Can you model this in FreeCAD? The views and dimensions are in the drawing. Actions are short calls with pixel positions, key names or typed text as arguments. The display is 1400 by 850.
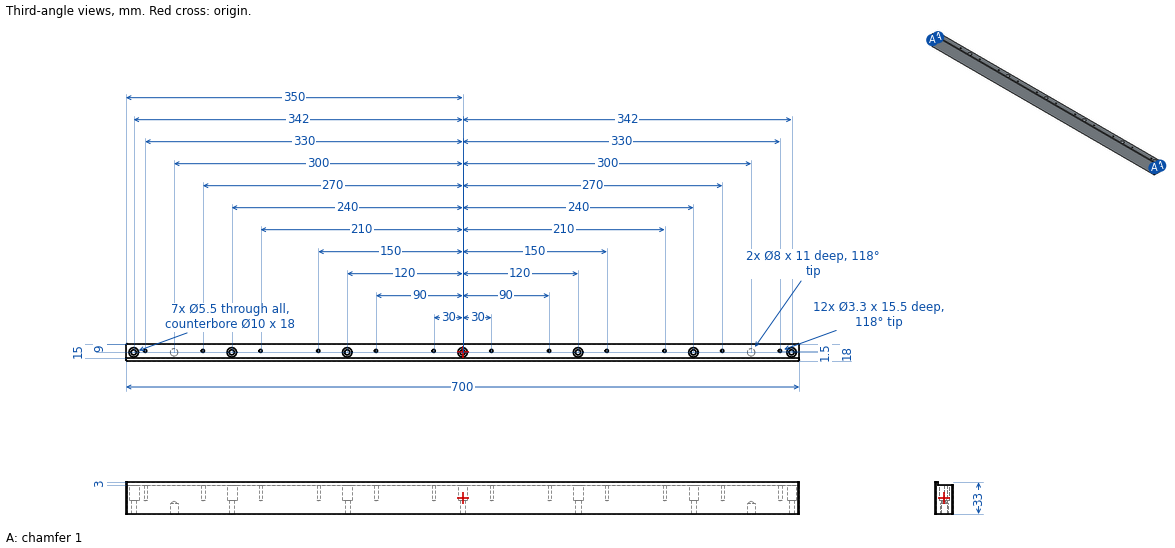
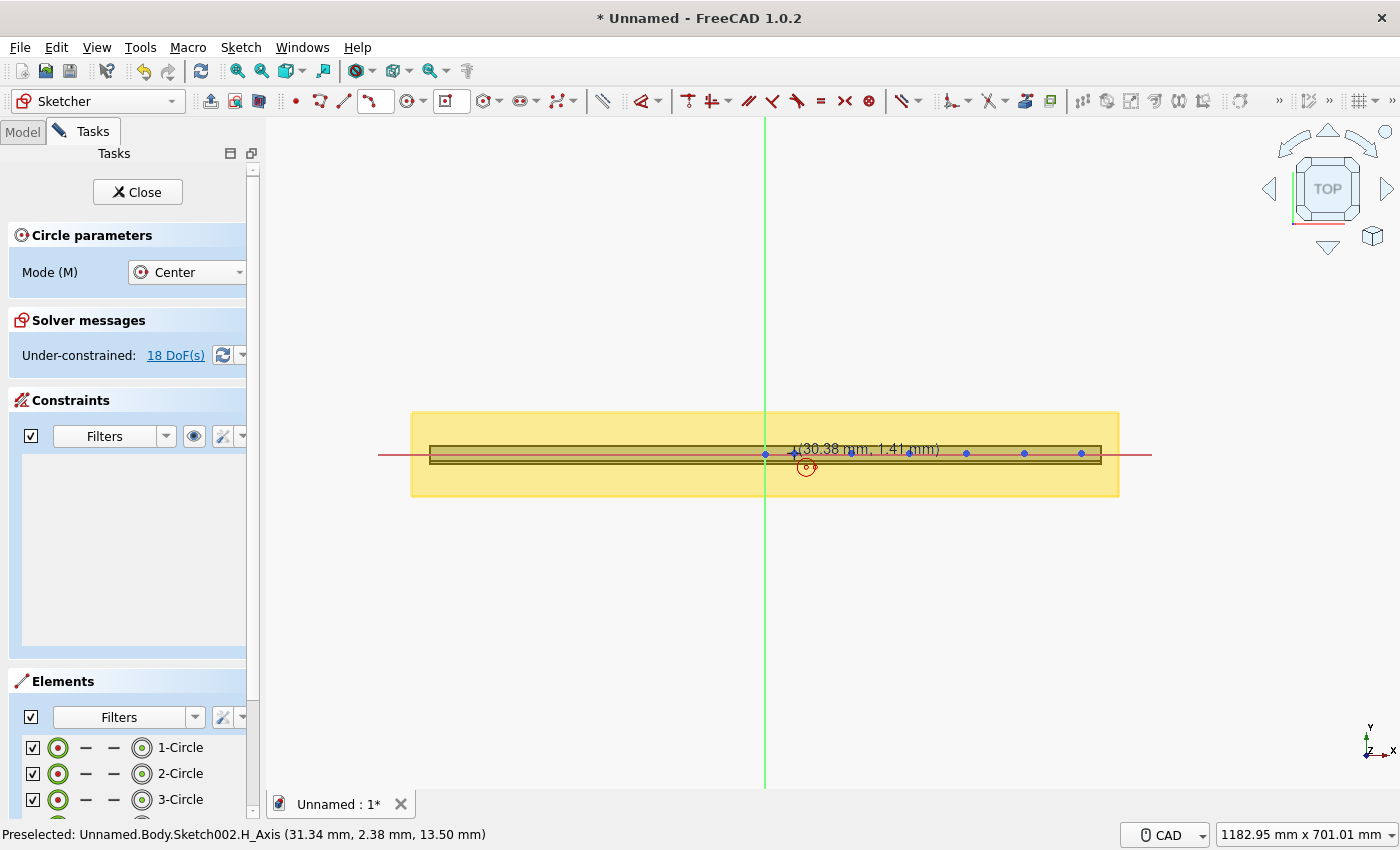
scroll(737, 453, up, 14)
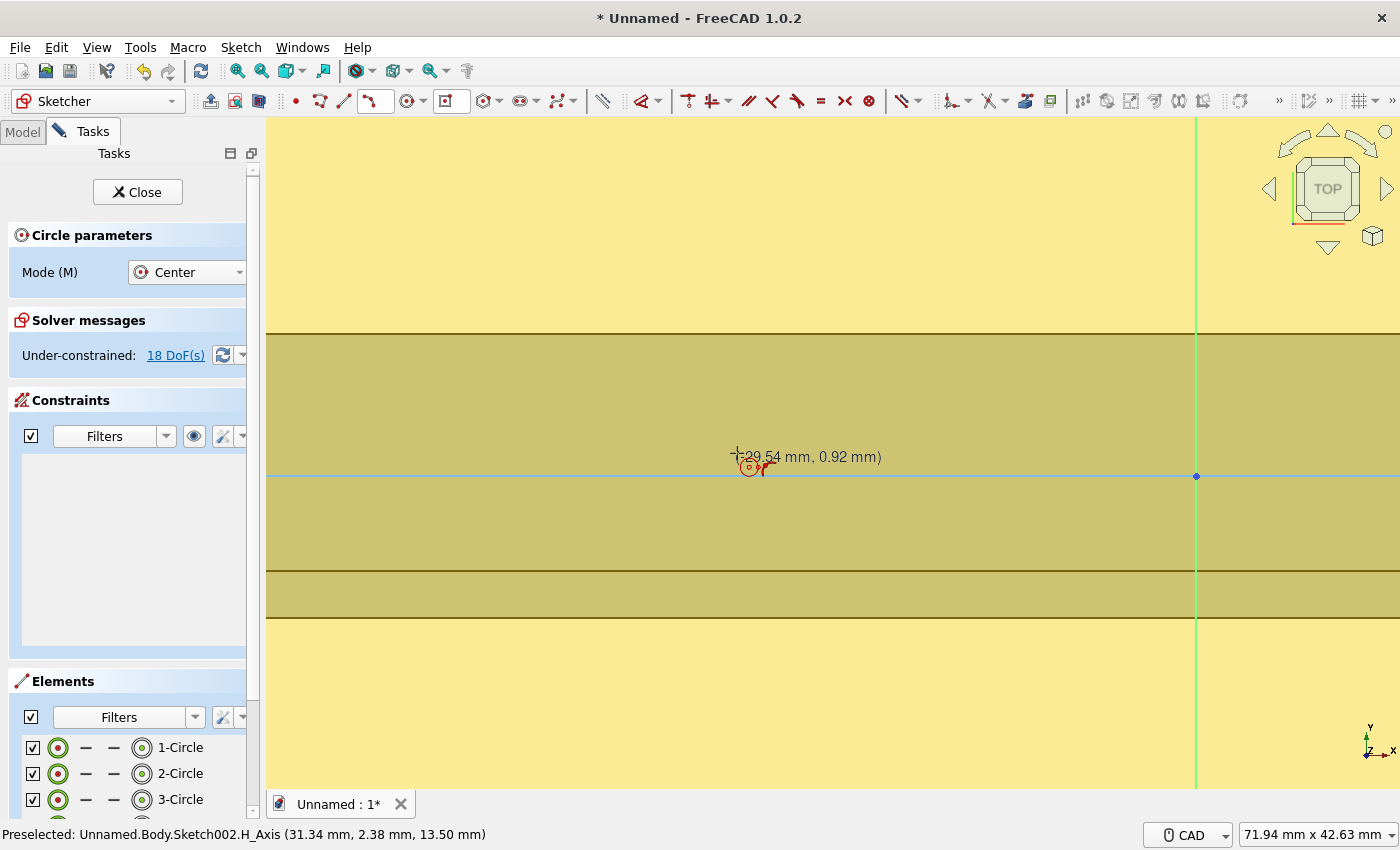
click(723, 453)
click(742, 434)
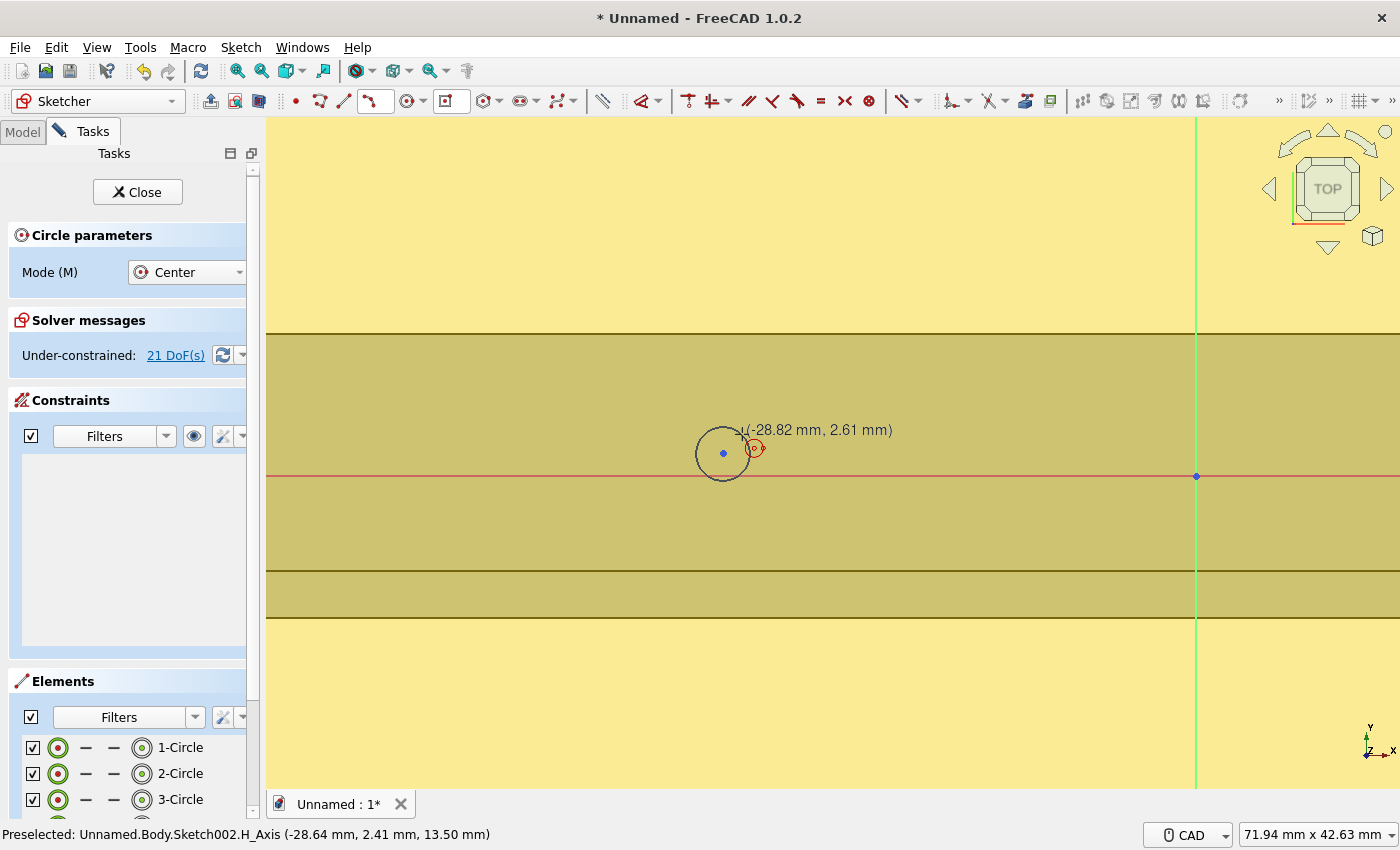
scroll(737, 453, down, 14)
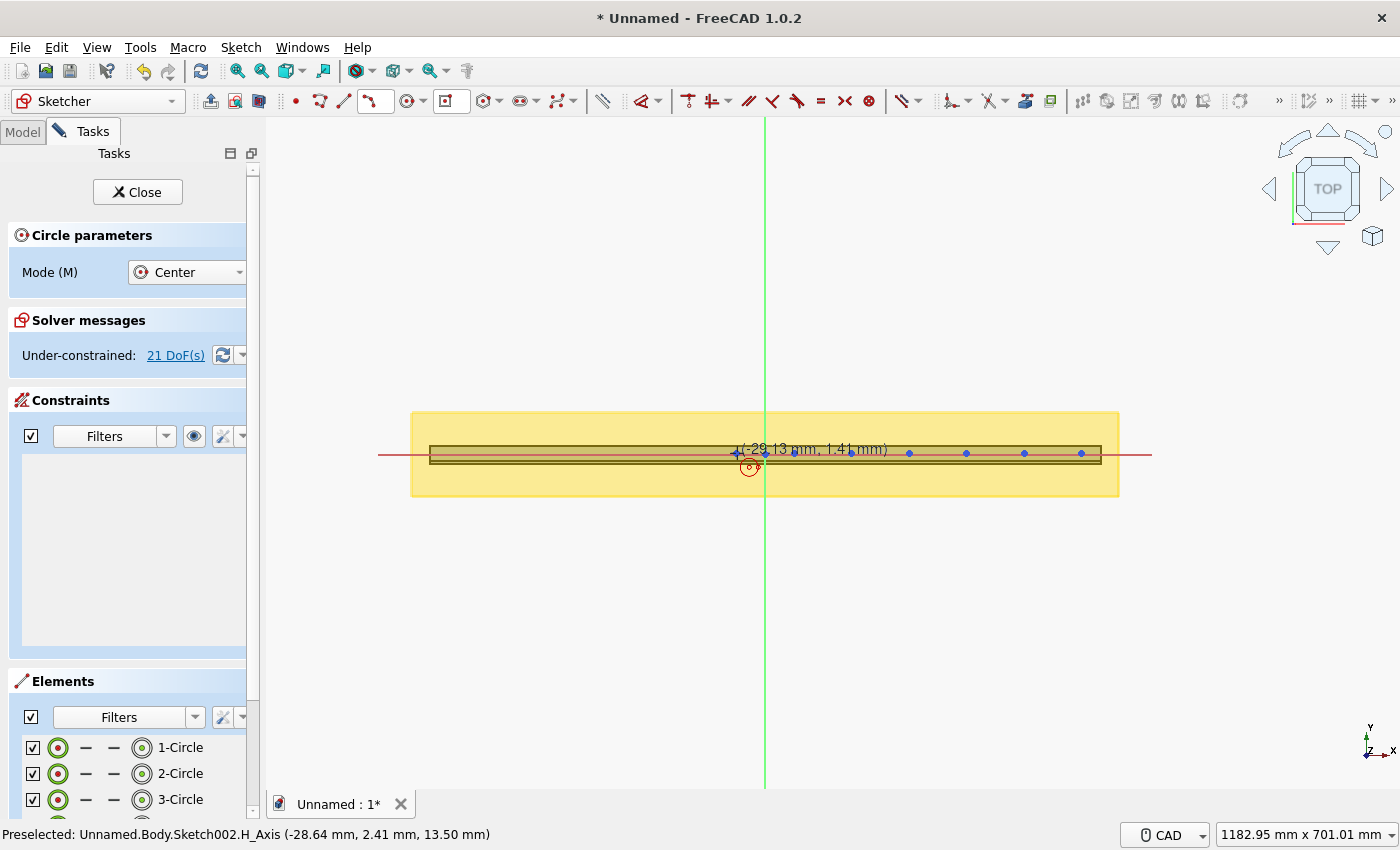
scroll(679, 453, up, 14)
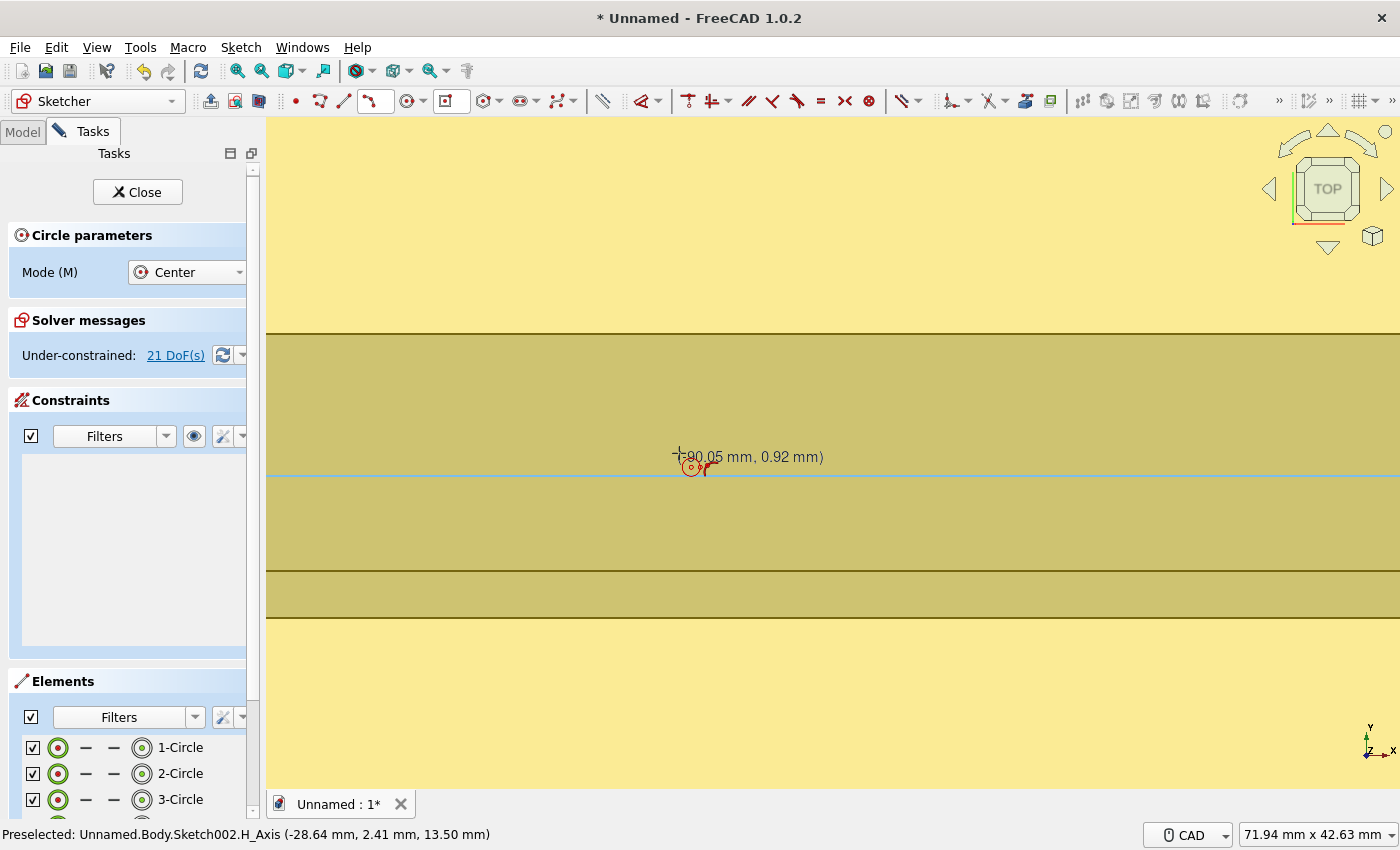
click(674, 453)
click(692, 434)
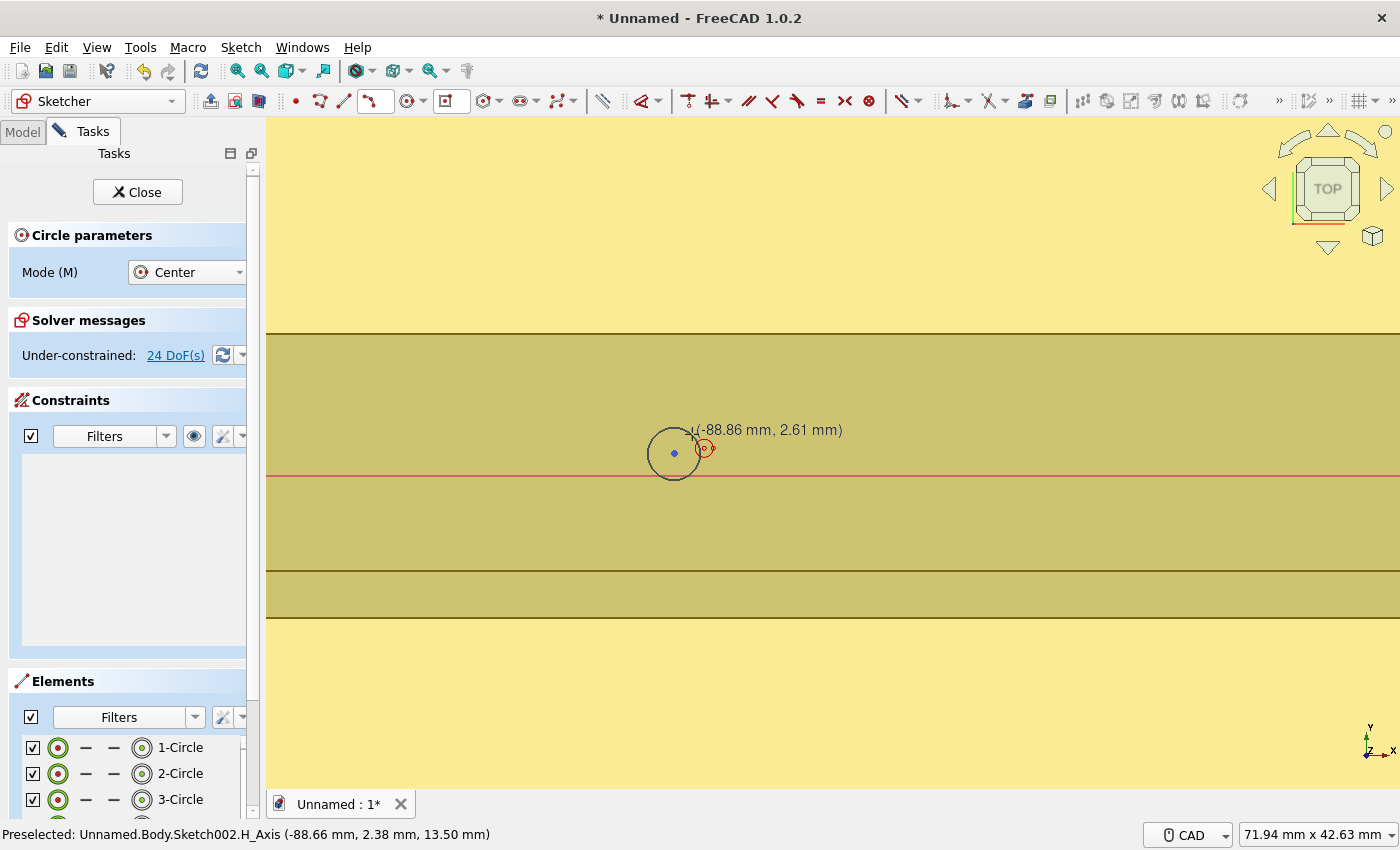
scroll(678, 453, down, 14)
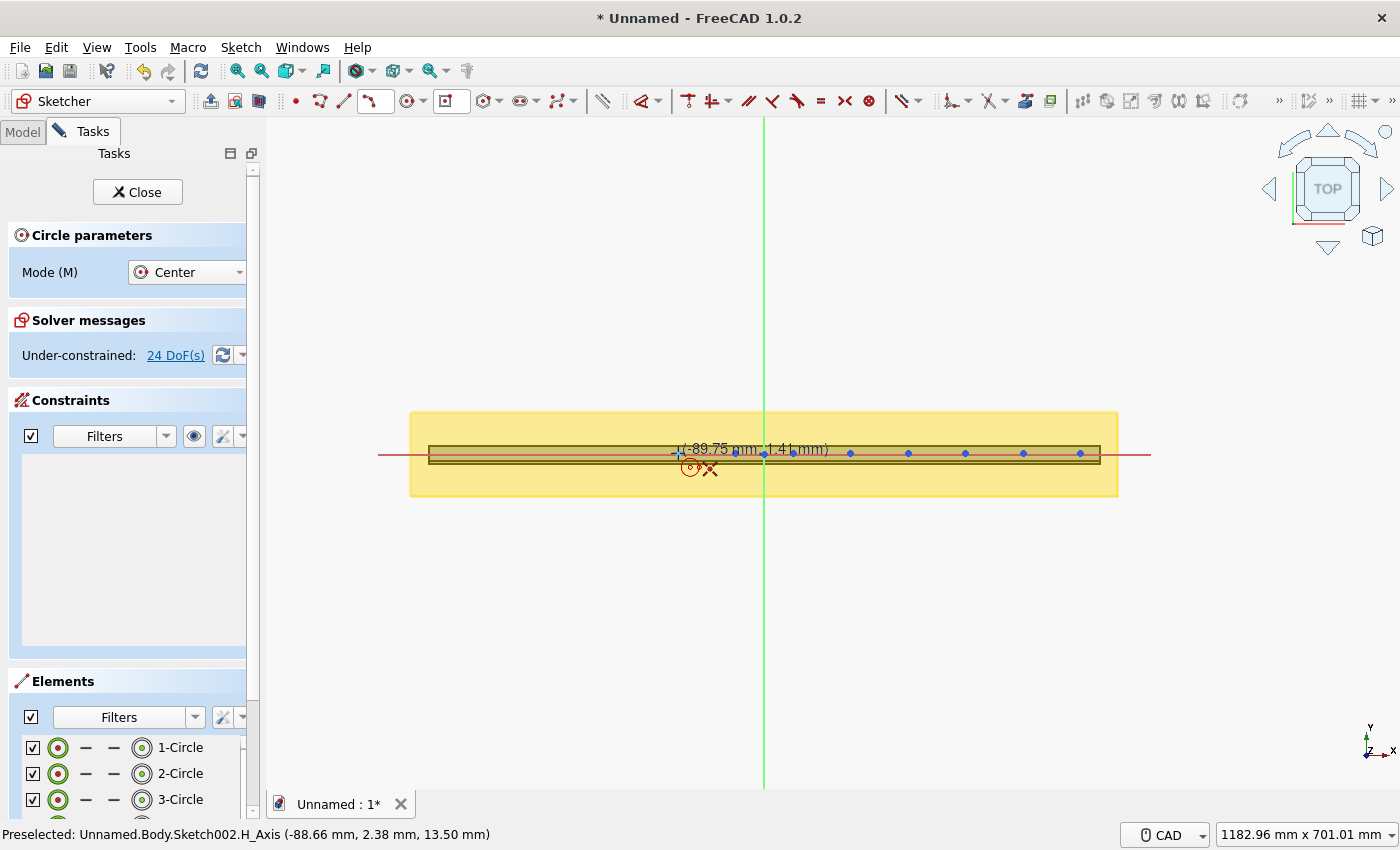
scroll(621, 453, up, 14)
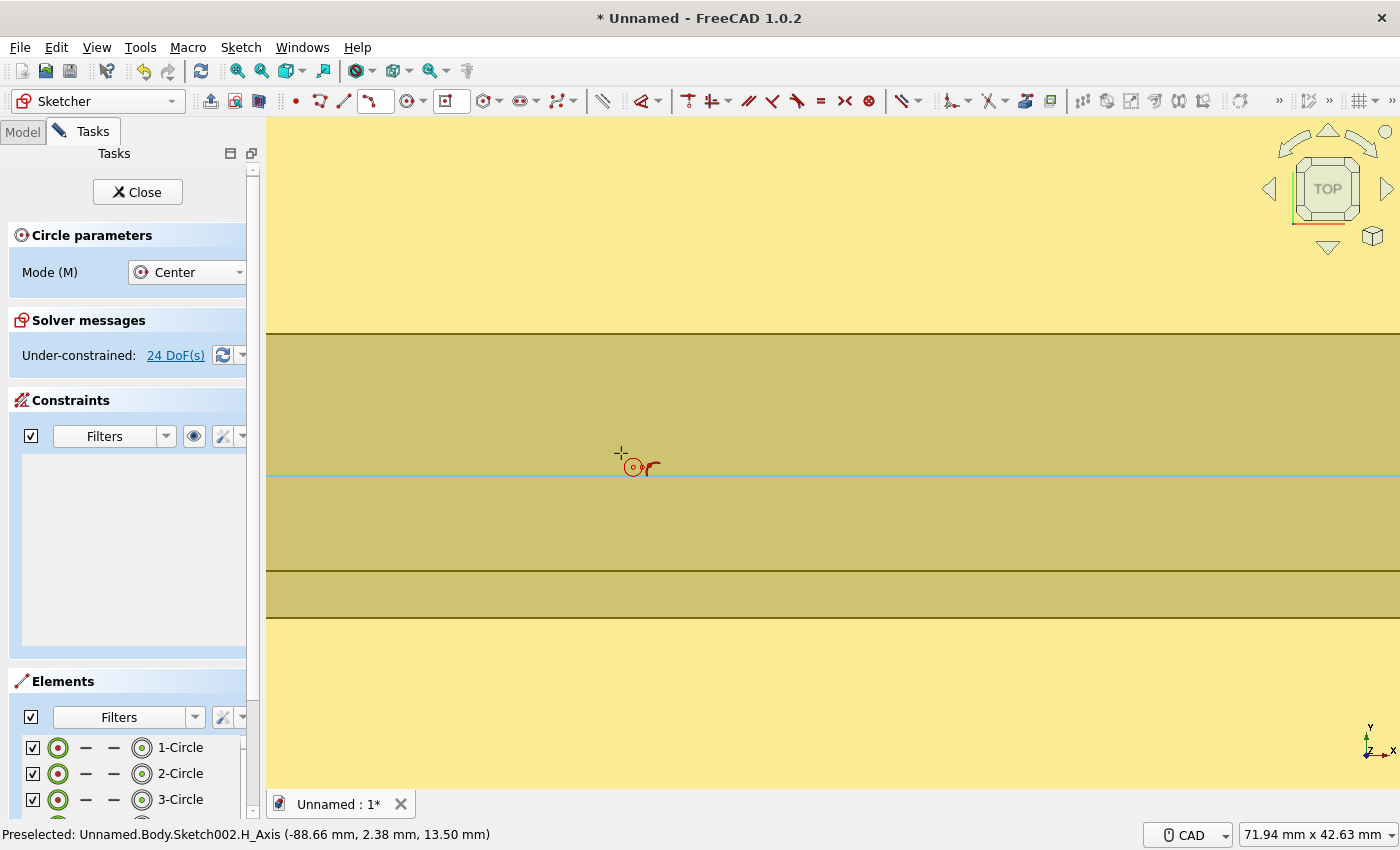
click(609, 453)
click(628, 434)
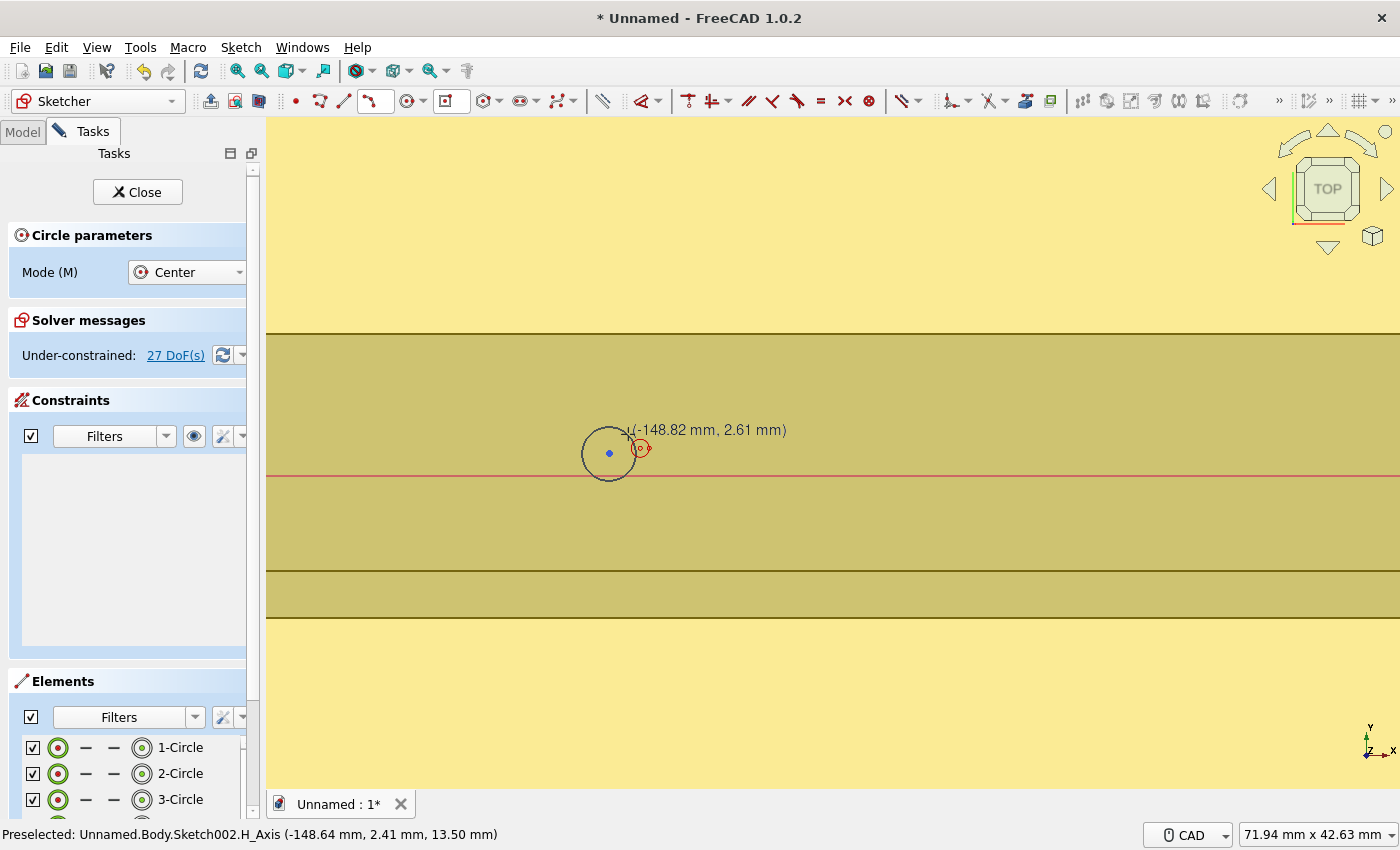
scroll(621, 453, down, 14)